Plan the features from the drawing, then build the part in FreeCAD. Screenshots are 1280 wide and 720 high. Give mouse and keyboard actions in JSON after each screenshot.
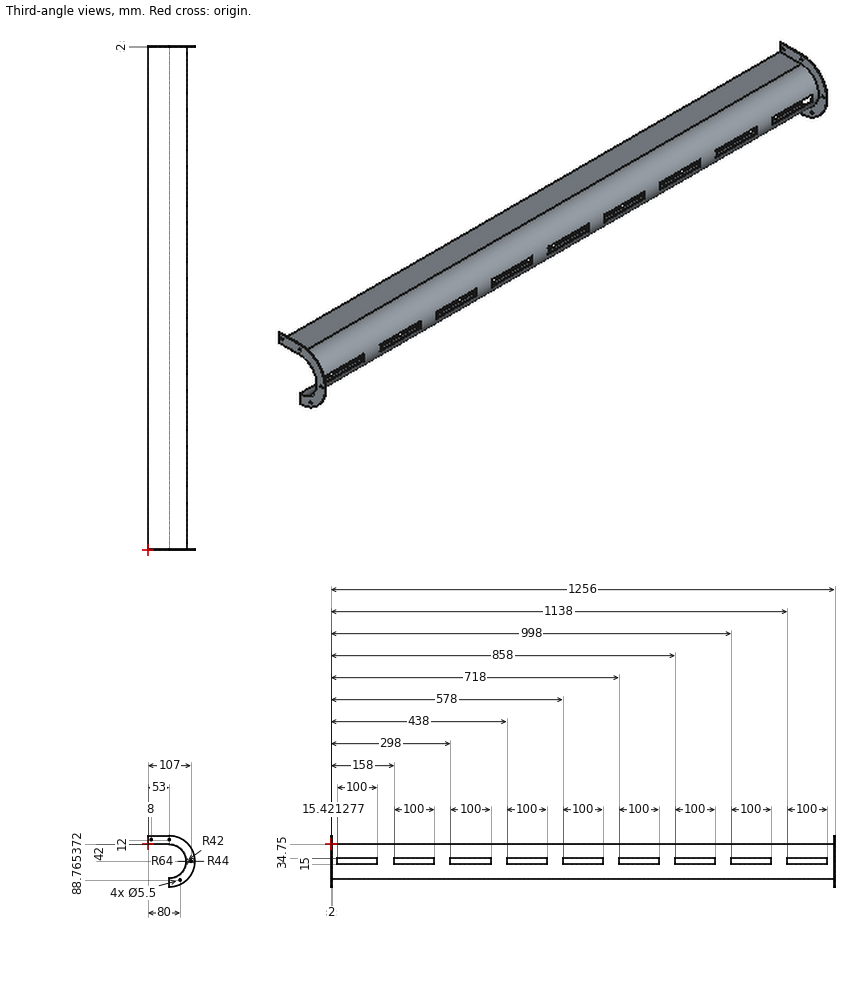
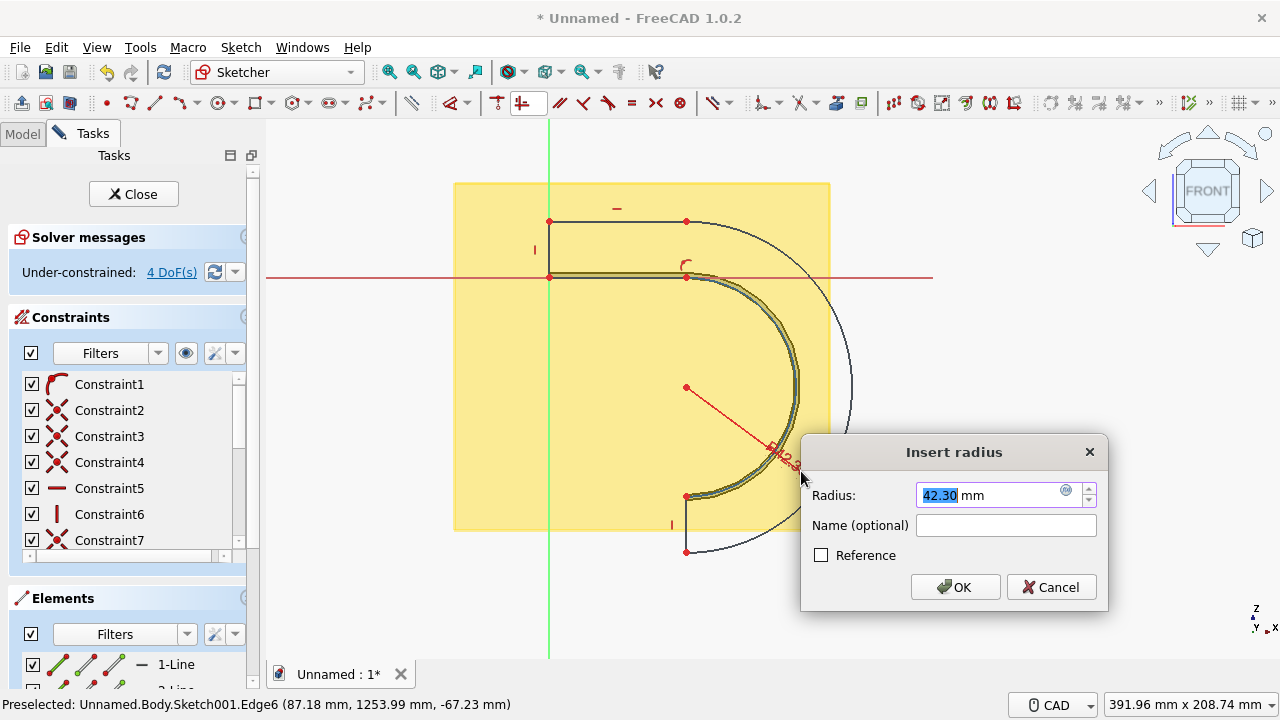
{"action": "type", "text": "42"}
{"action": "key", "text": "Return"}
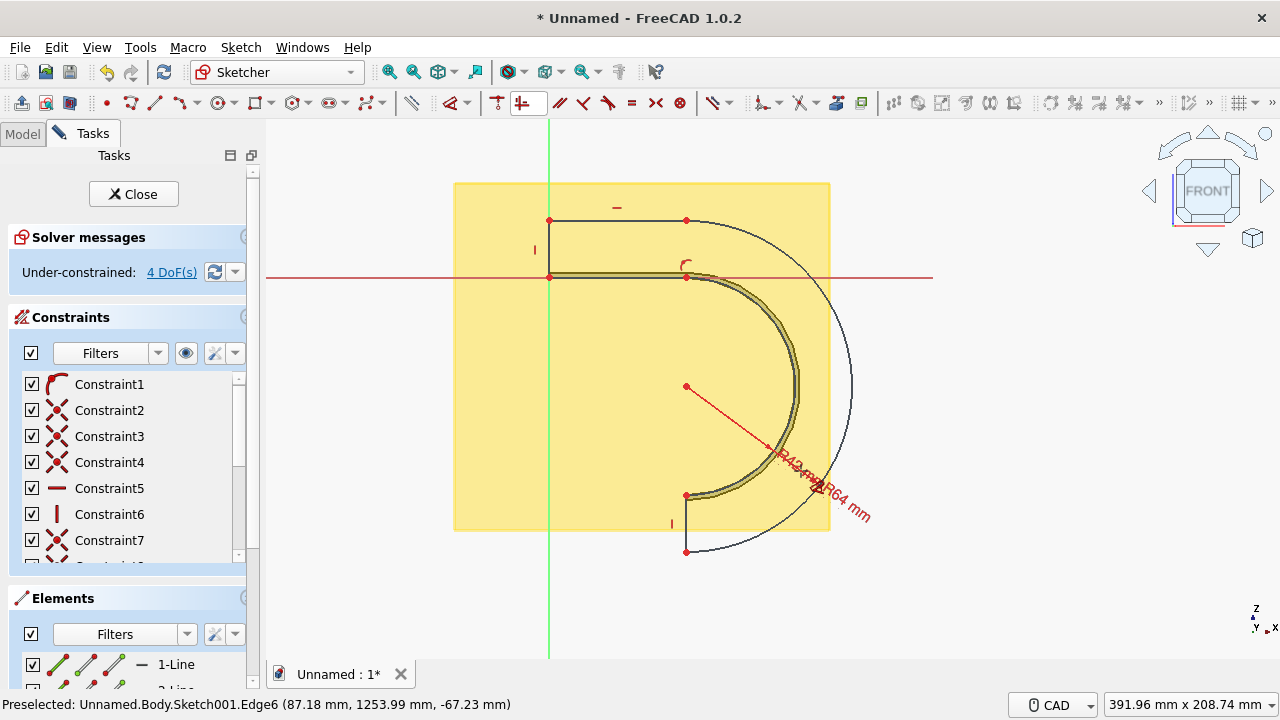
{"action": "left_click", "coordinate": [645, 278]}
{"action": "left_click", "coordinate": [618, 244]}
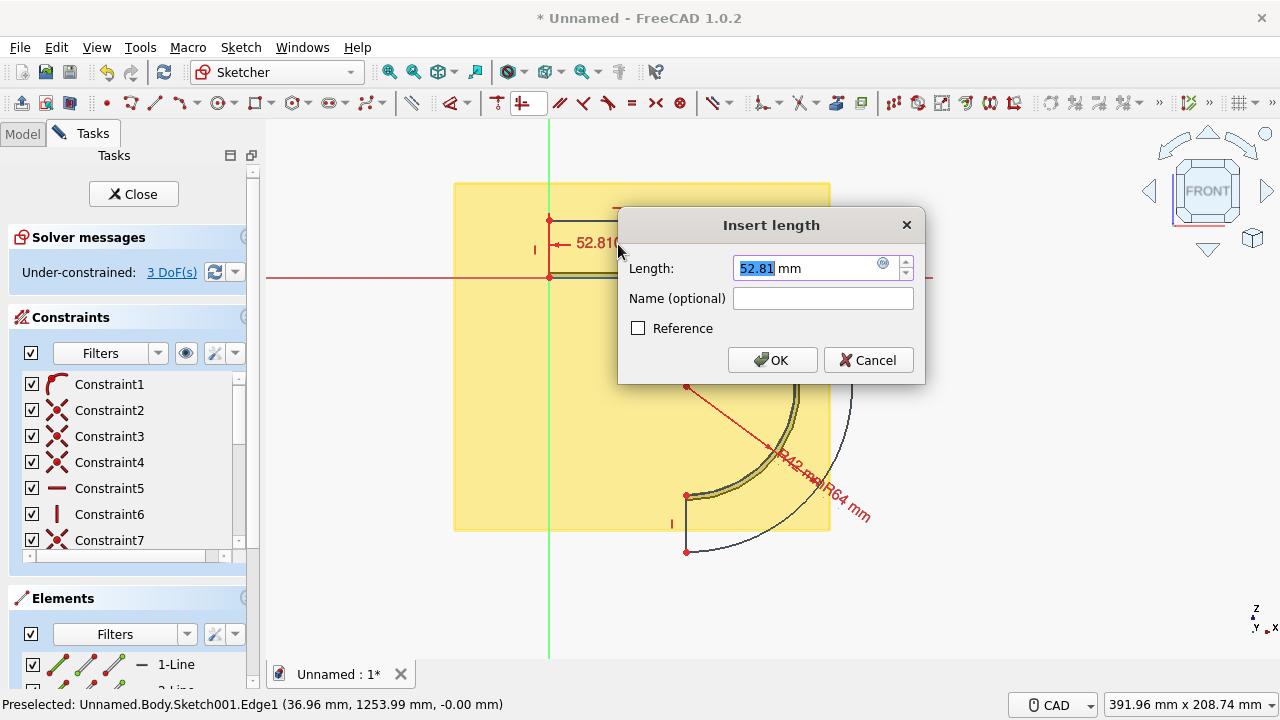
{"action": "type", "text": "53"}
{"action": "key", "text": "Return"}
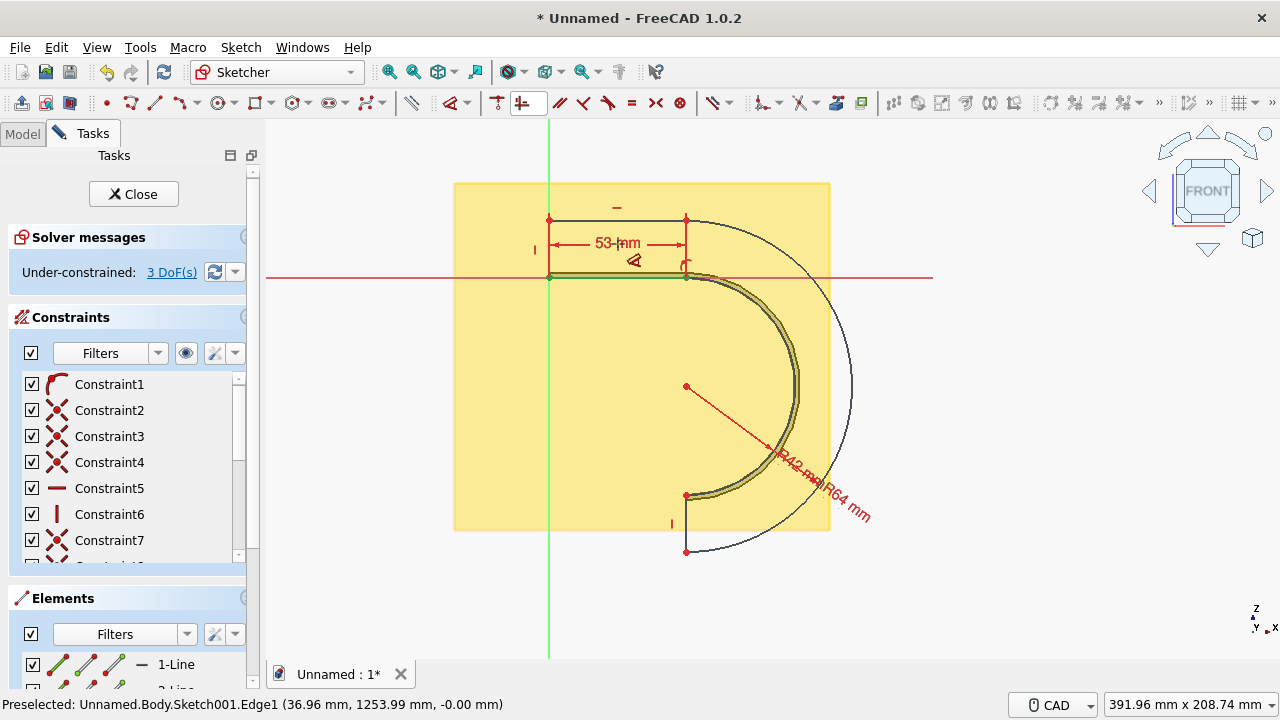
{"action": "left_click", "coordinate": [590, 221]}
{"action": "left_click", "coordinate": [618, 187]}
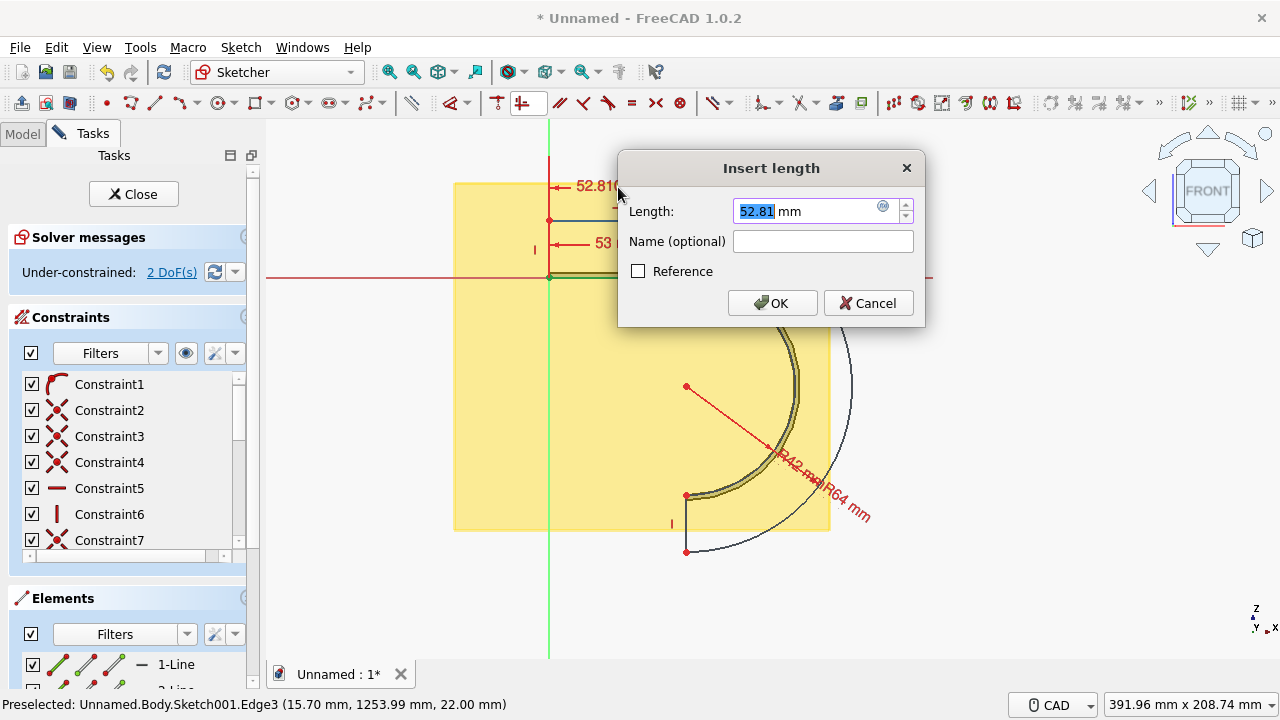
{"action": "type", "text": "53"}
{"action": "key", "text": "Return"}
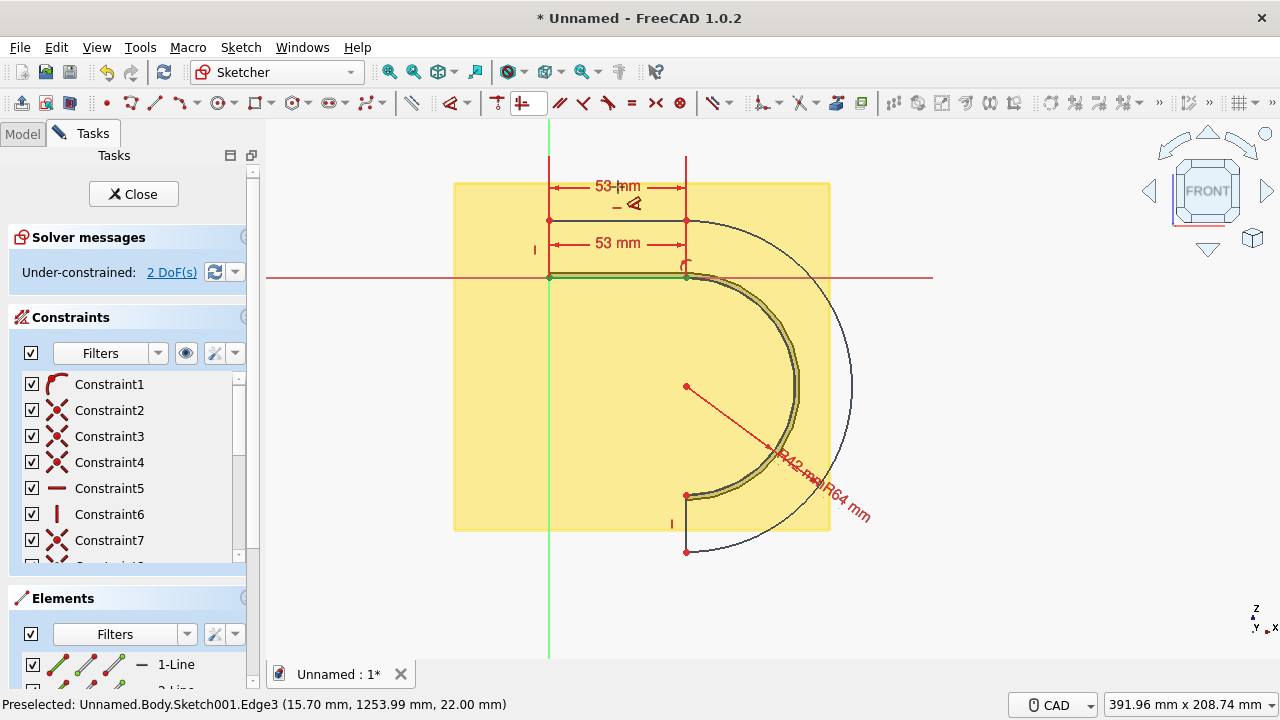
{"action": "left_click", "coordinate": [686, 552]}
{"action": "left_click", "coordinate": [618, 586]}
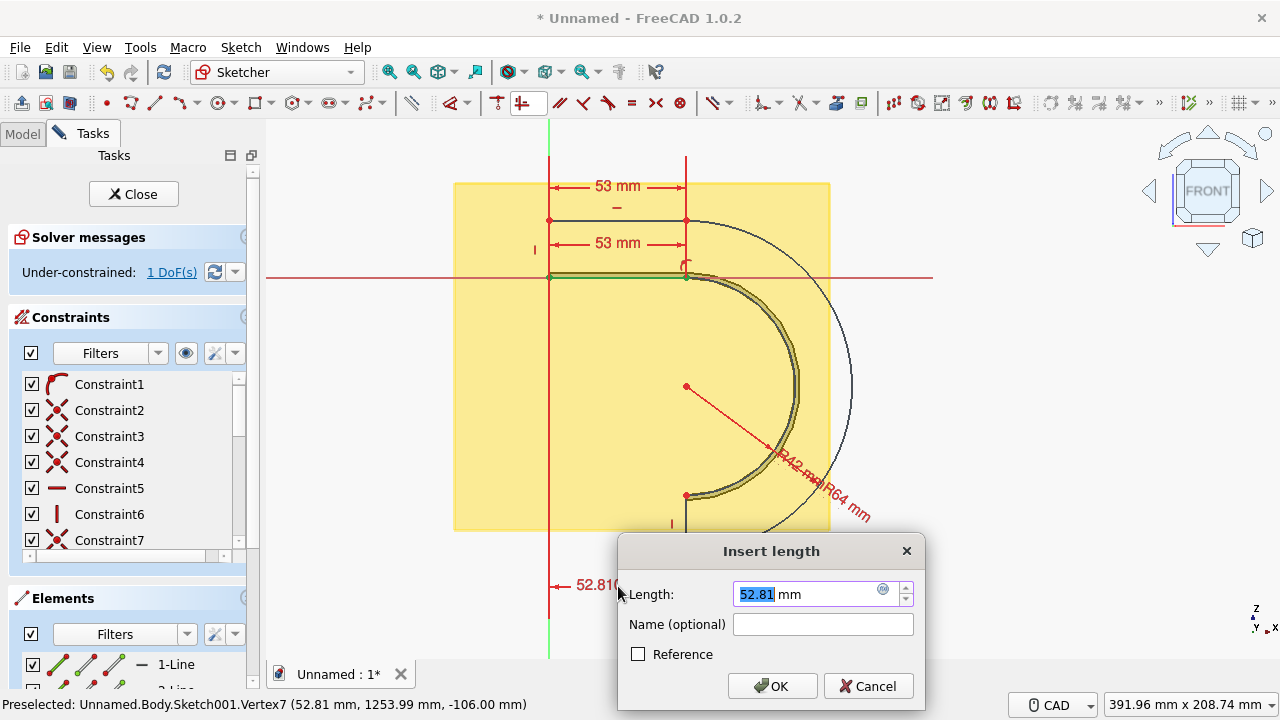
{"action": "type", "text": "53"}
{"action": "key", "text": "Return"}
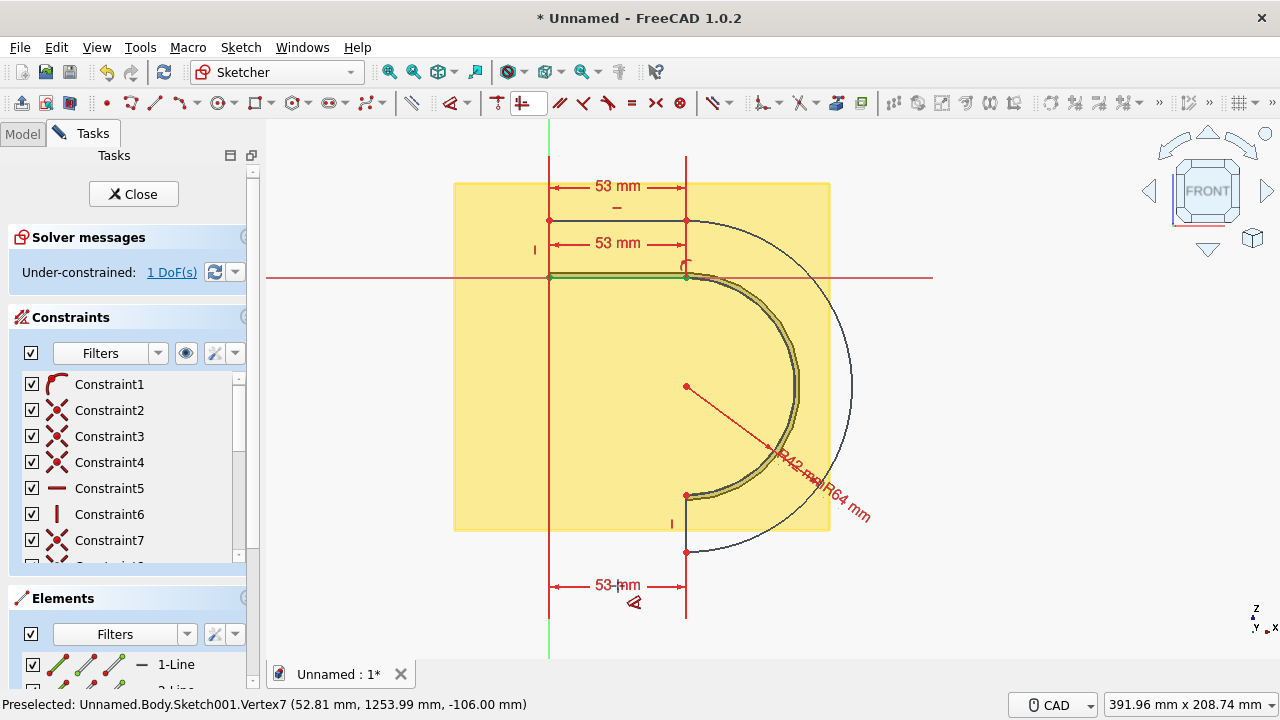
{"action": "left_click", "coordinate": [686, 386]}
{"action": "left_click", "coordinate": [618, 420]}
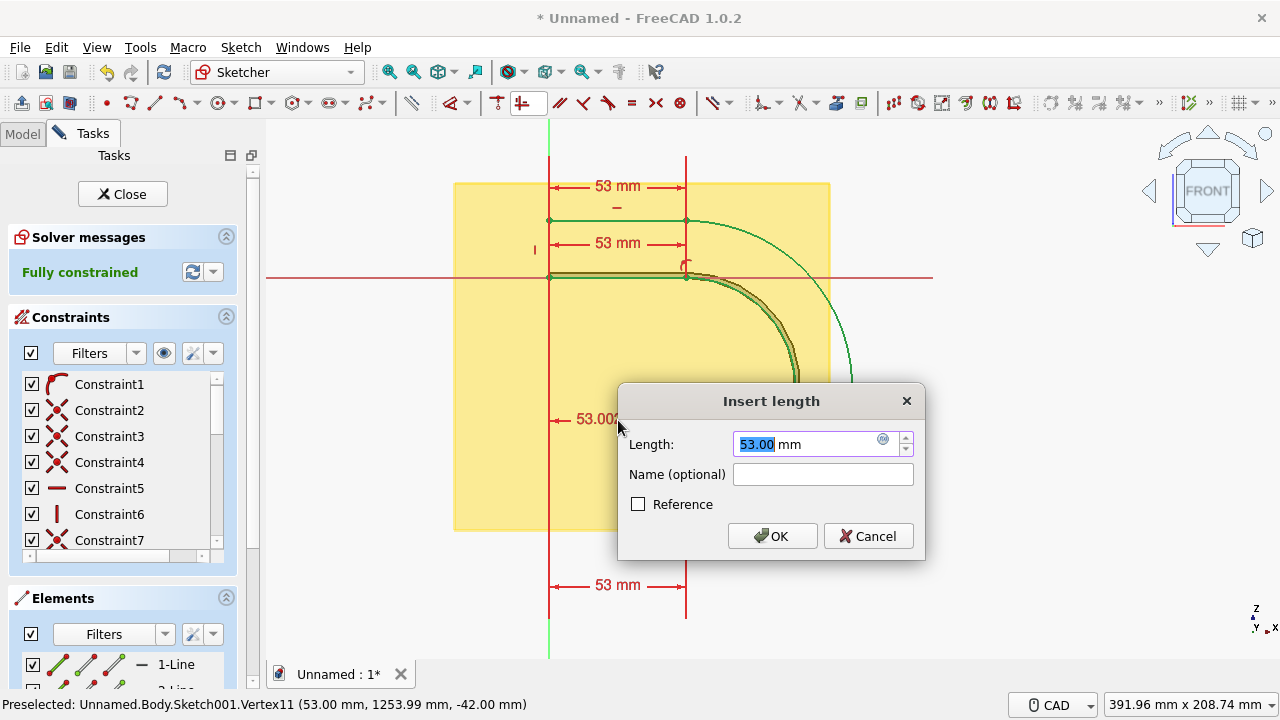
{"action": "type", "text": "53"}
{"action": "key", "text": "Return"}
{"action": "key", "text": "Escape"}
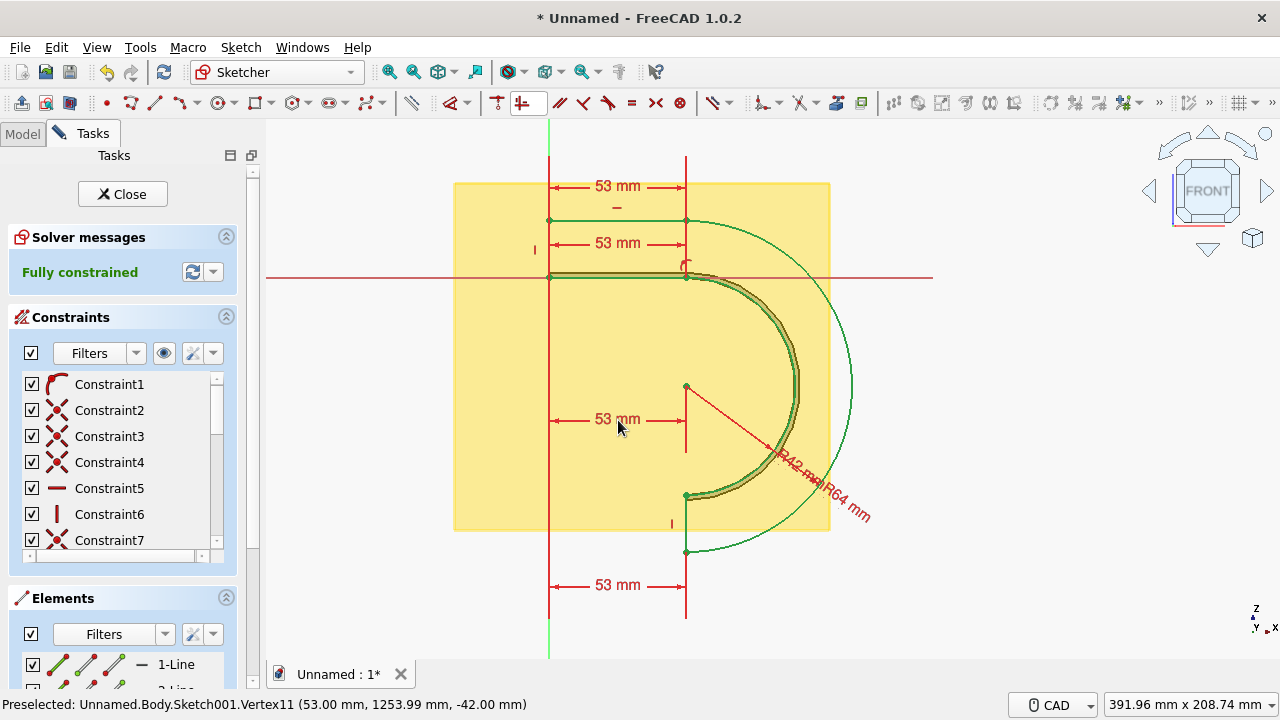
{"action": "left_click", "coordinate": [123, 194]}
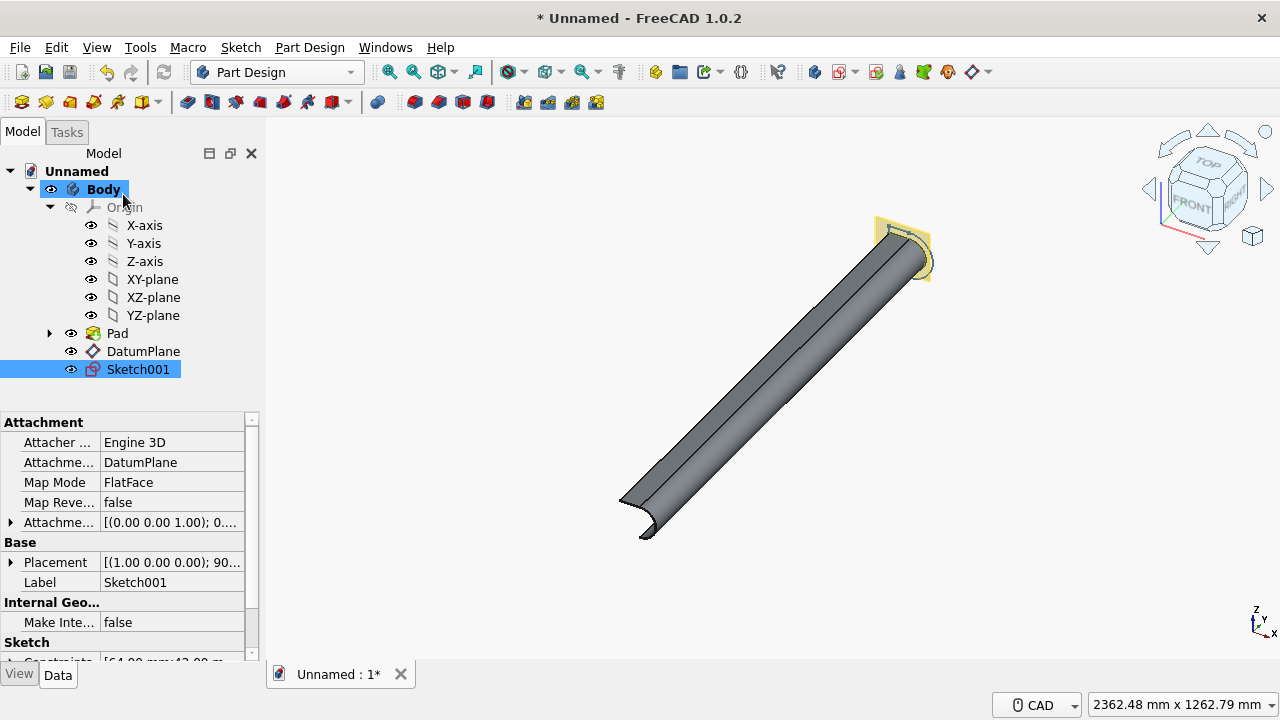
{"action": "left_click", "coordinate": [22, 102]}